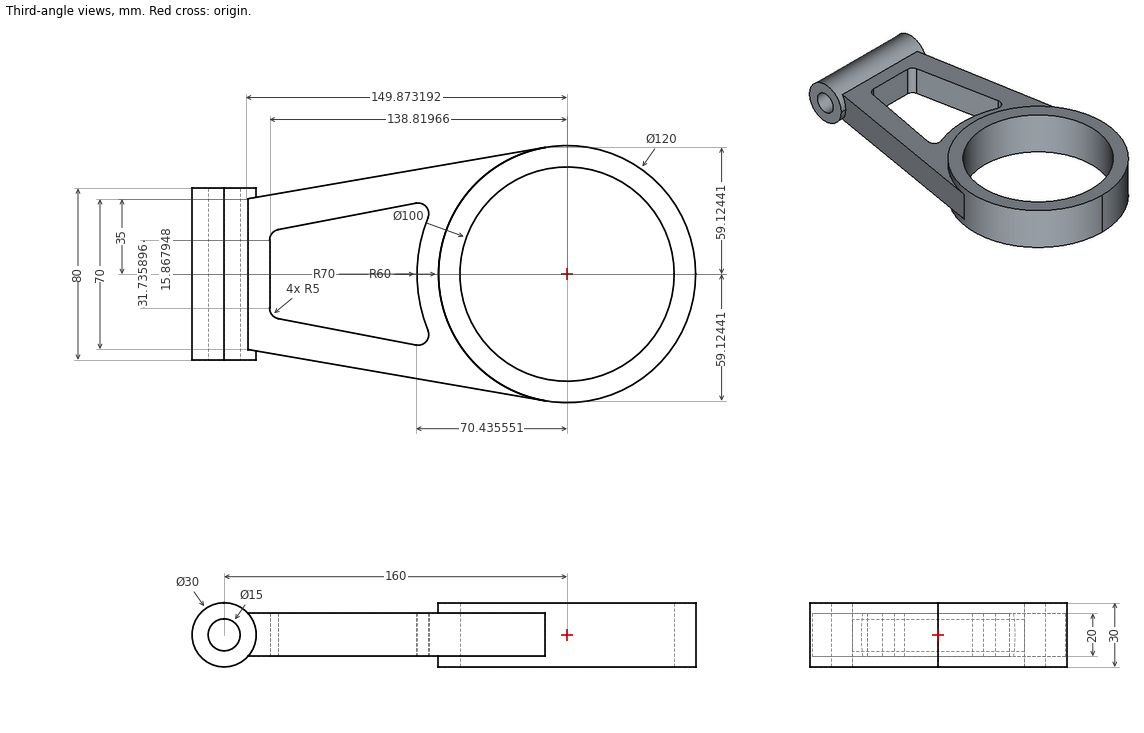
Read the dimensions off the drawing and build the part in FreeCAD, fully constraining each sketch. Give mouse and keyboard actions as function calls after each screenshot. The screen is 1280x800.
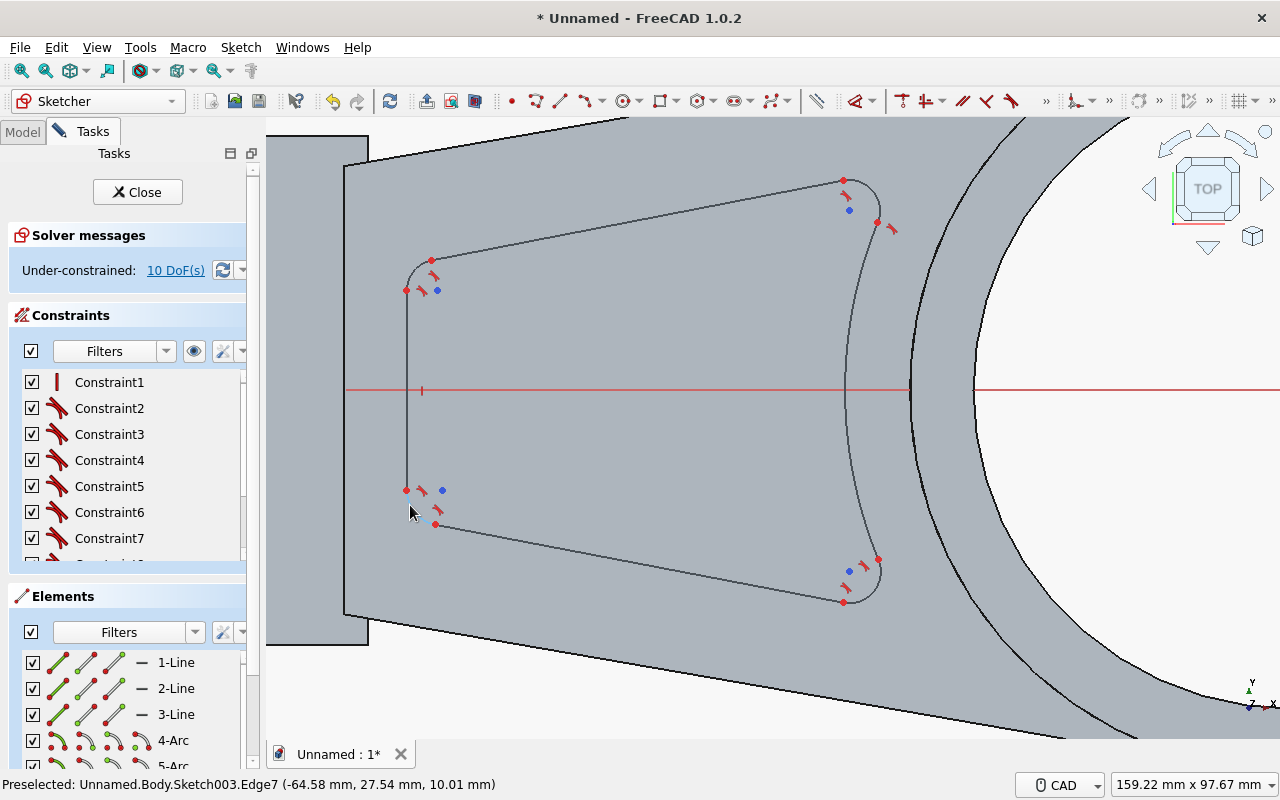
click(410, 504)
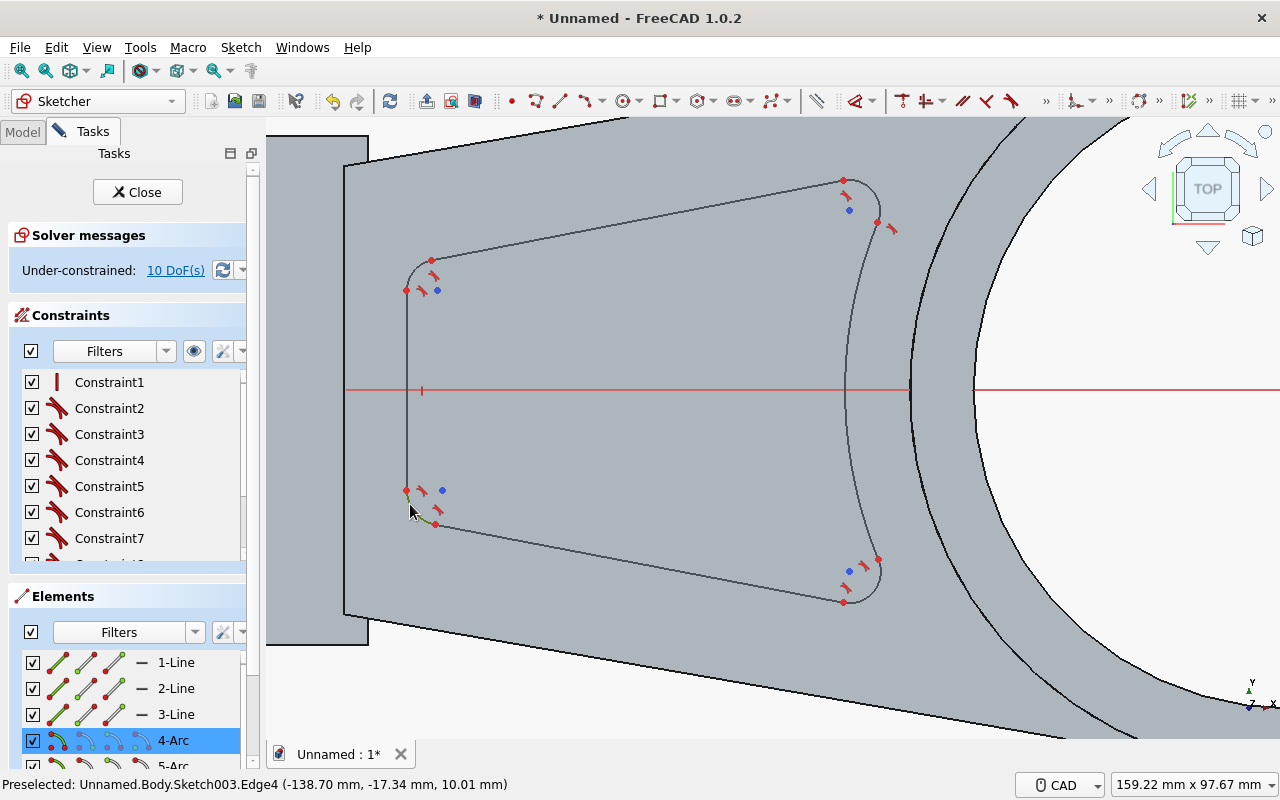
click(863, 600)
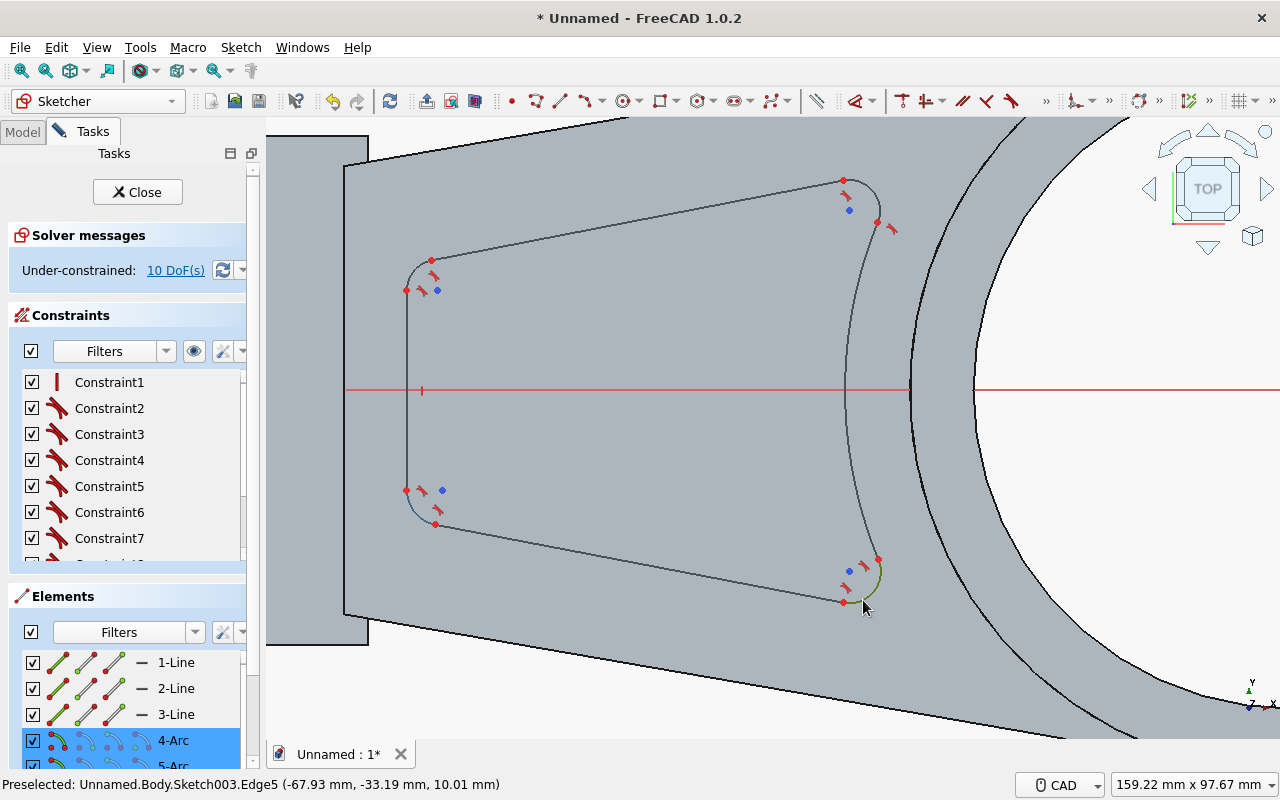
click(879, 203)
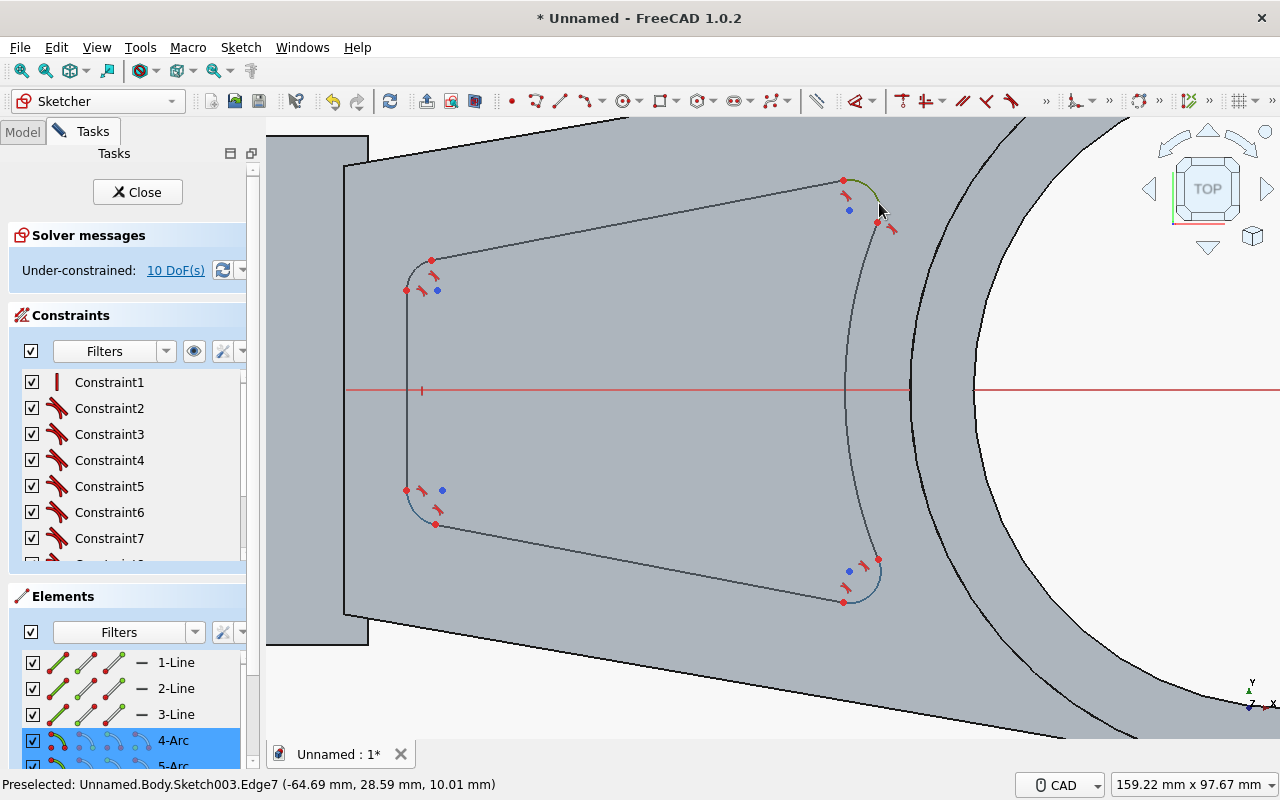
click(420, 265)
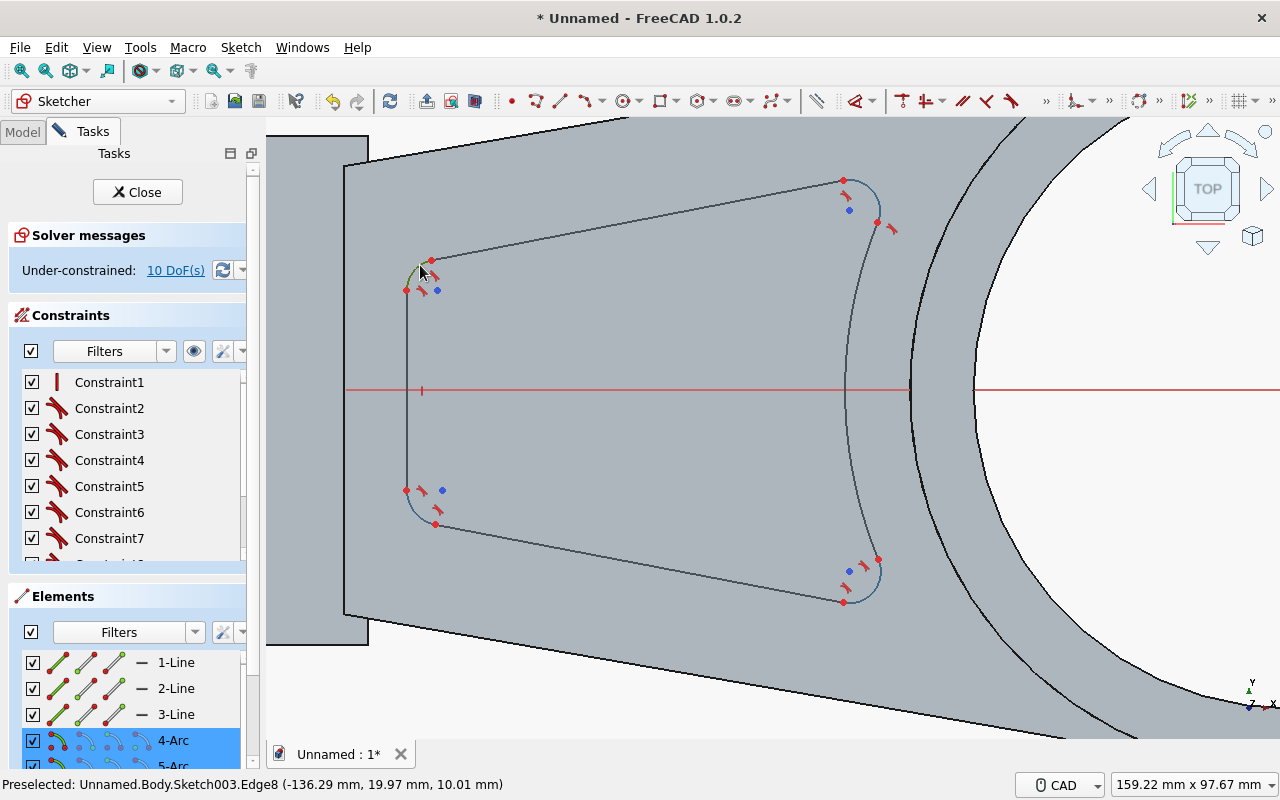
key(e)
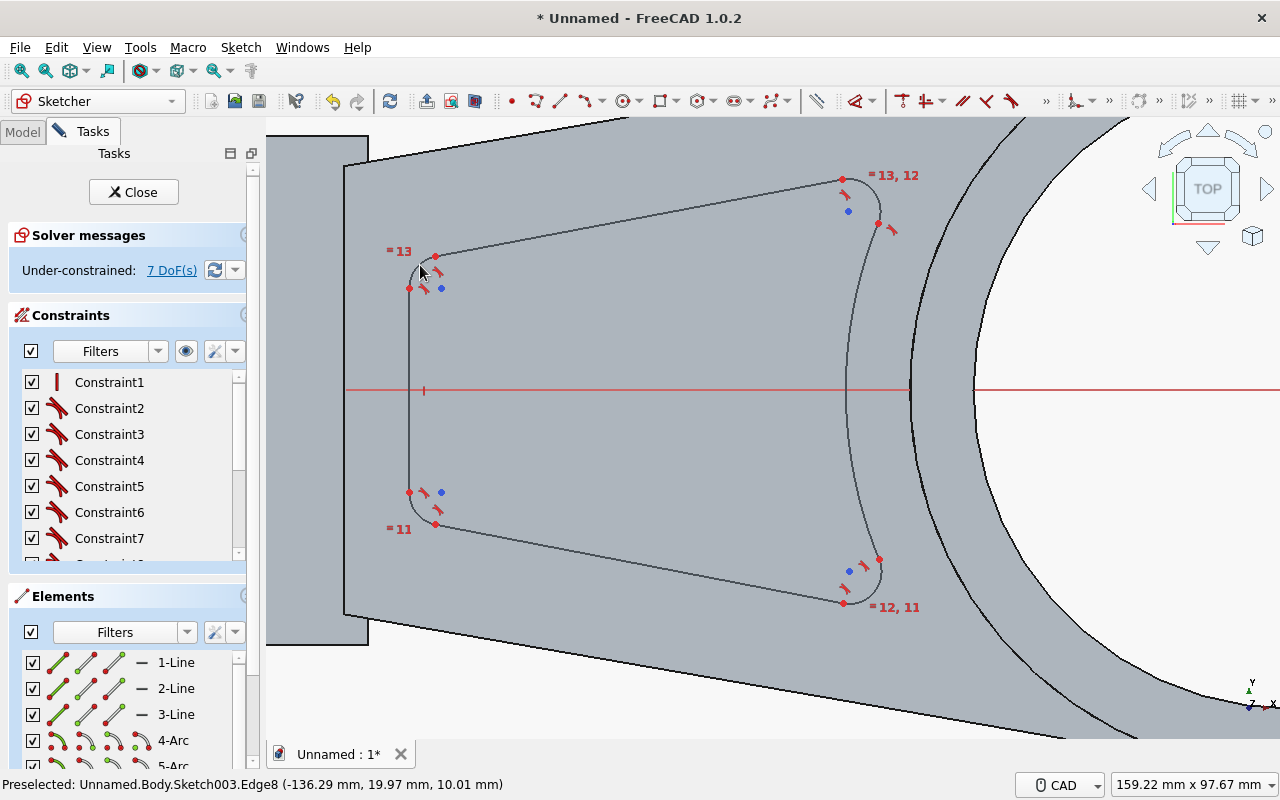
click(856, 102)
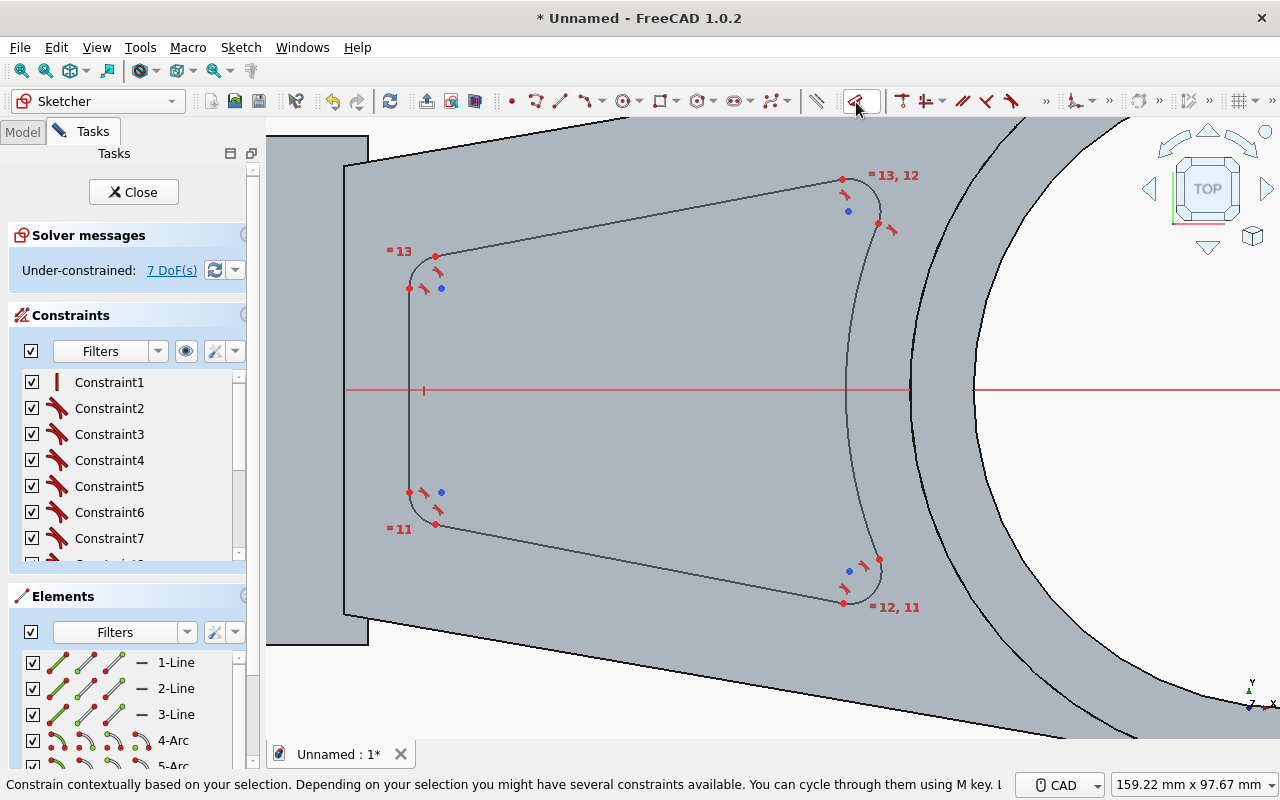
scroll(412, 506, up, 2)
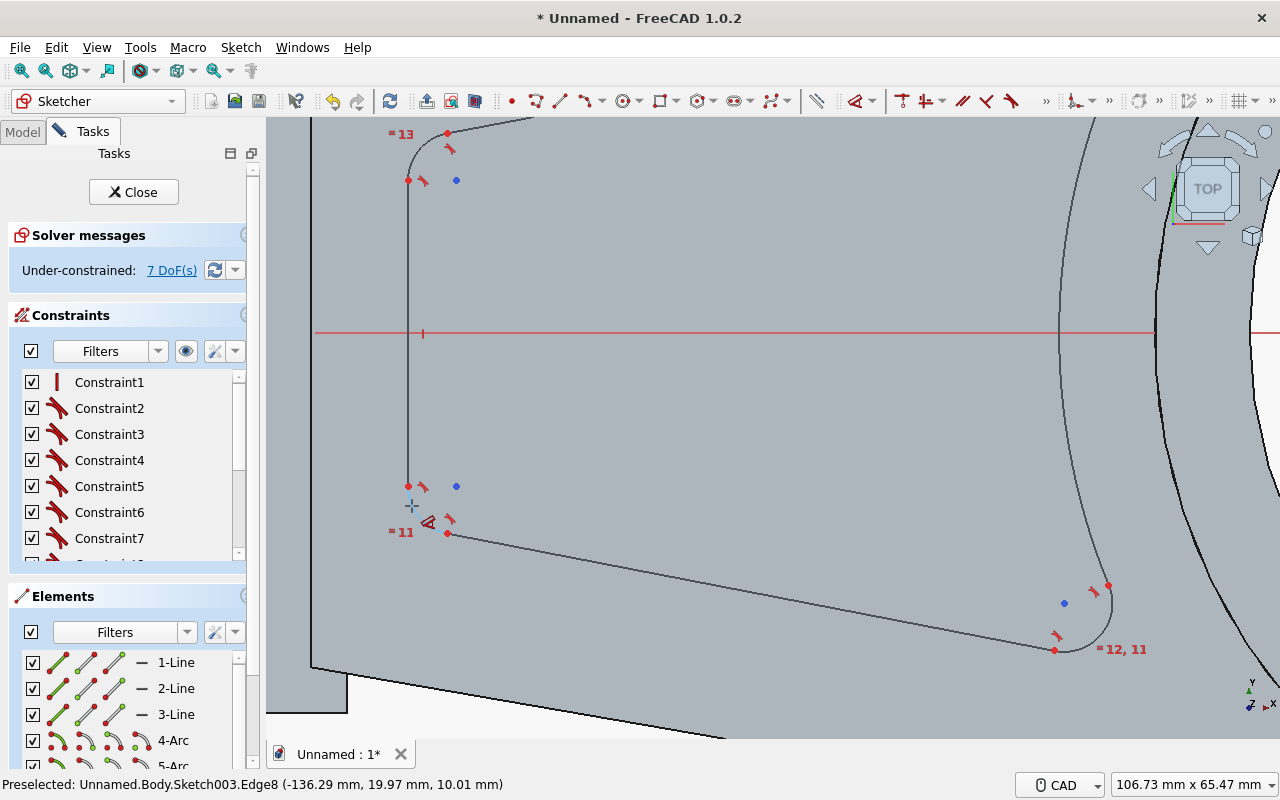
click(412, 506)
click(383, 519)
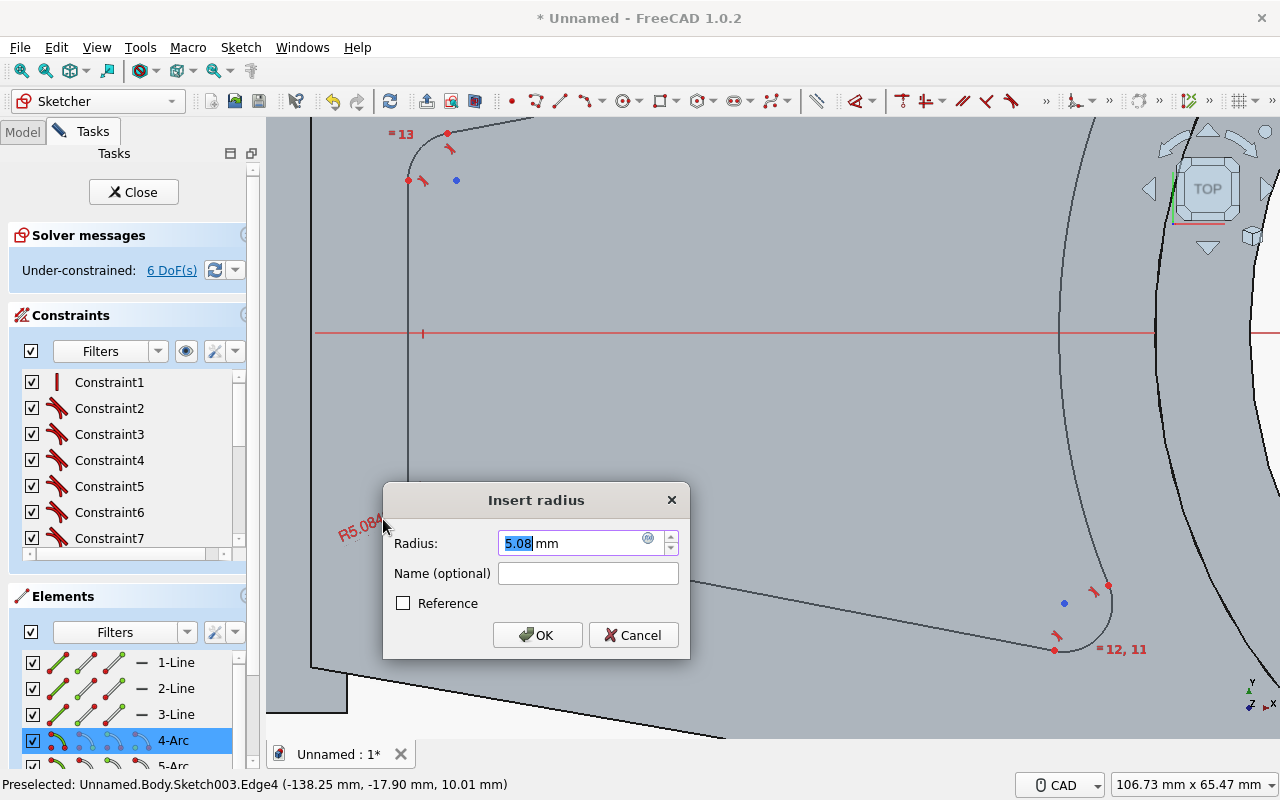
text(5)
key(Return)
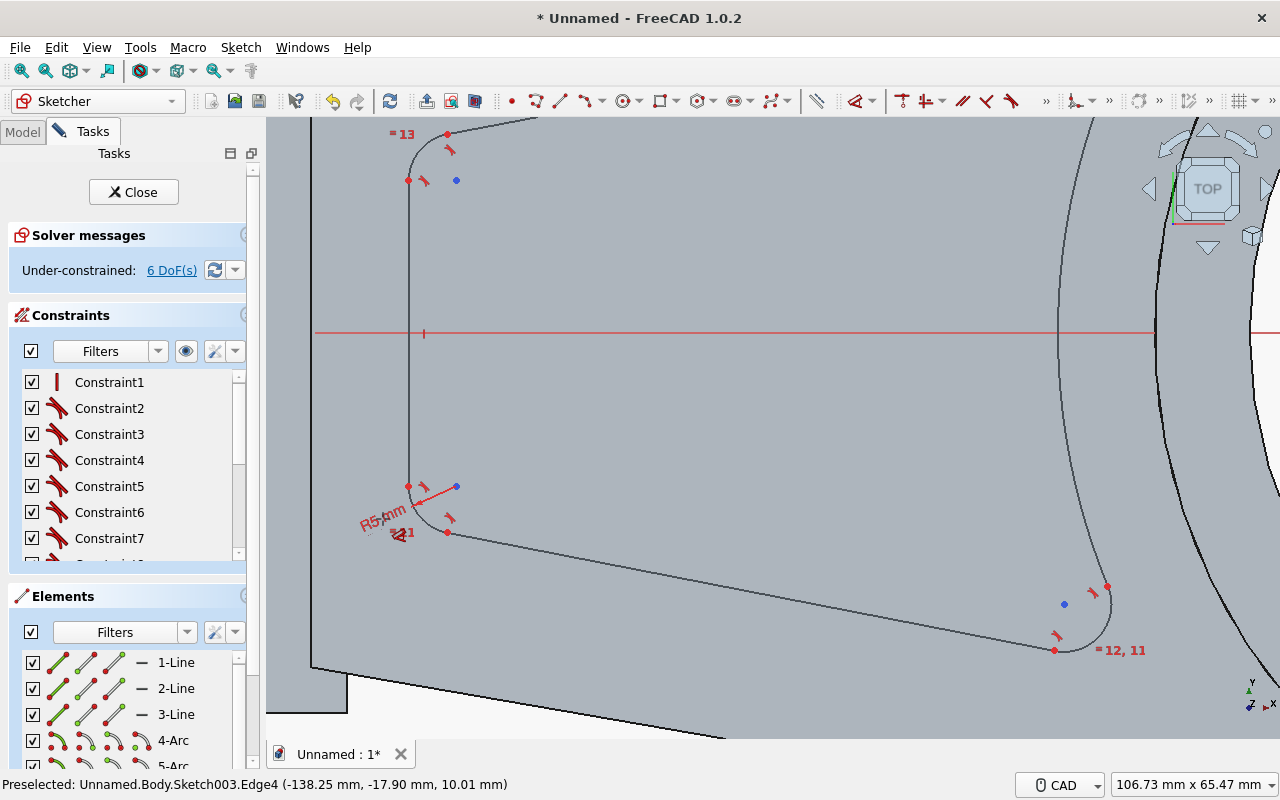
click(1066, 233)
click(1034, 228)